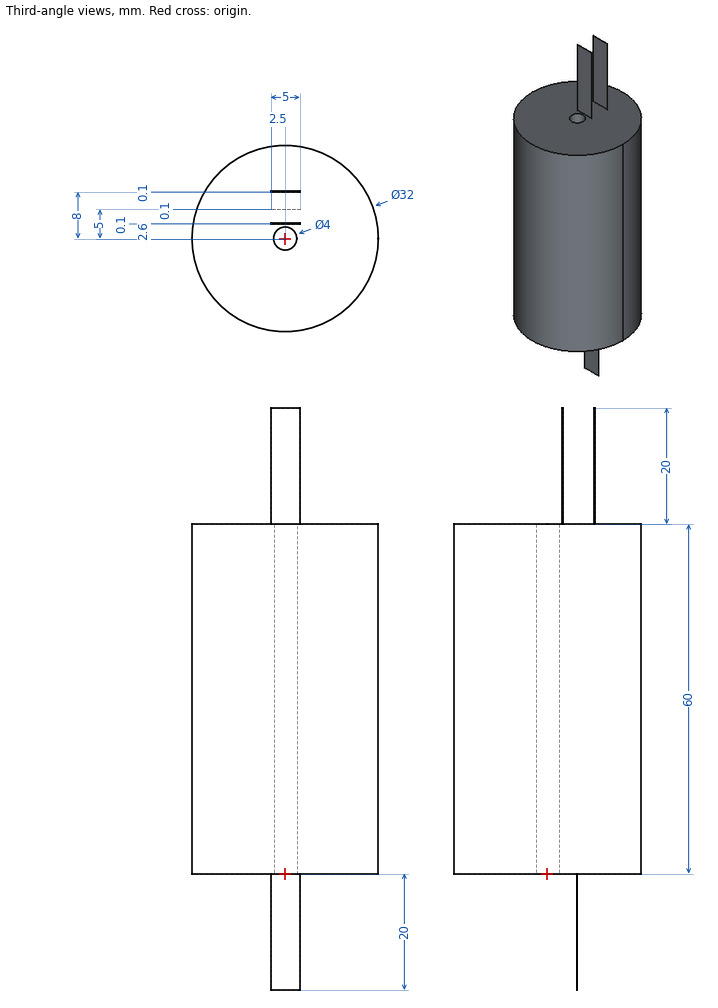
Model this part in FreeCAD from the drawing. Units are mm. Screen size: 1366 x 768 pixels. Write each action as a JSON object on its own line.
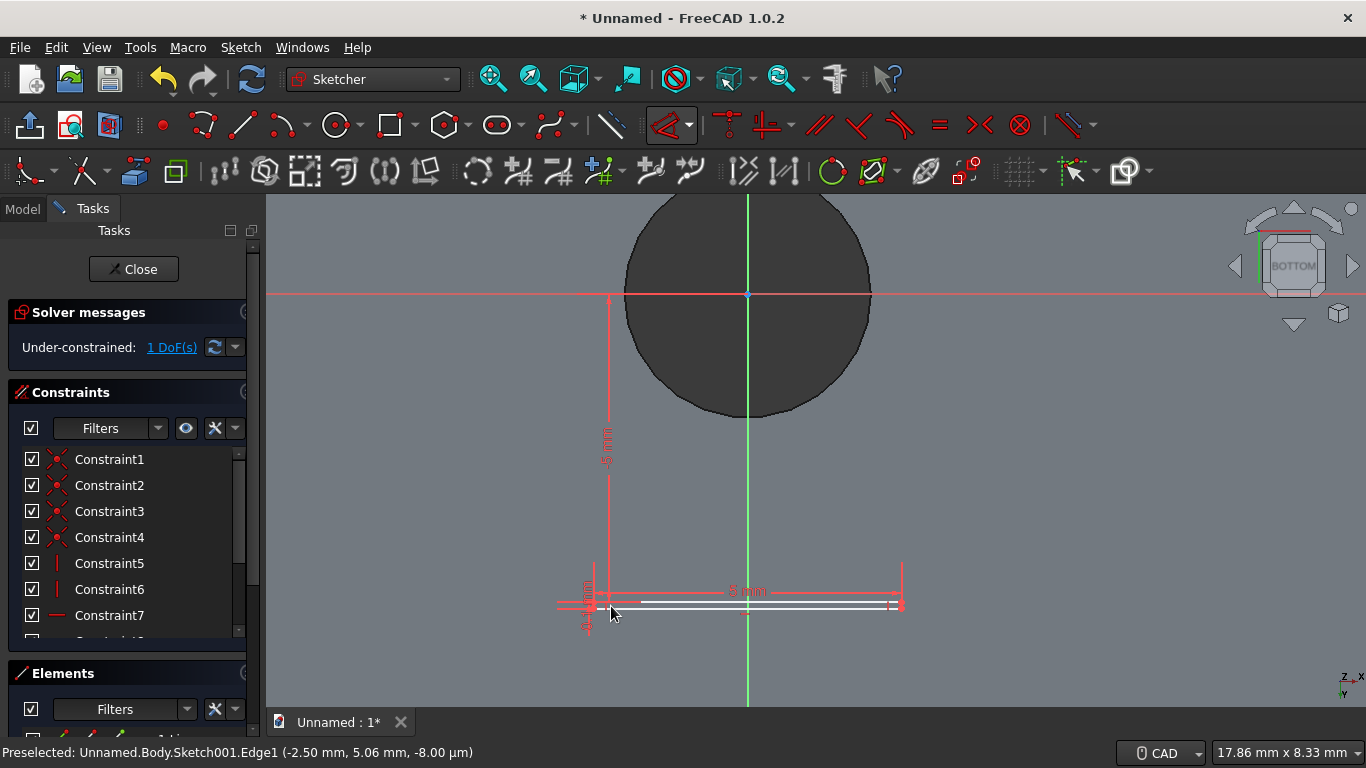
{"action": "scroll", "coordinate": [594, 602], "scroll_direction": "up", "scroll_amount": 4}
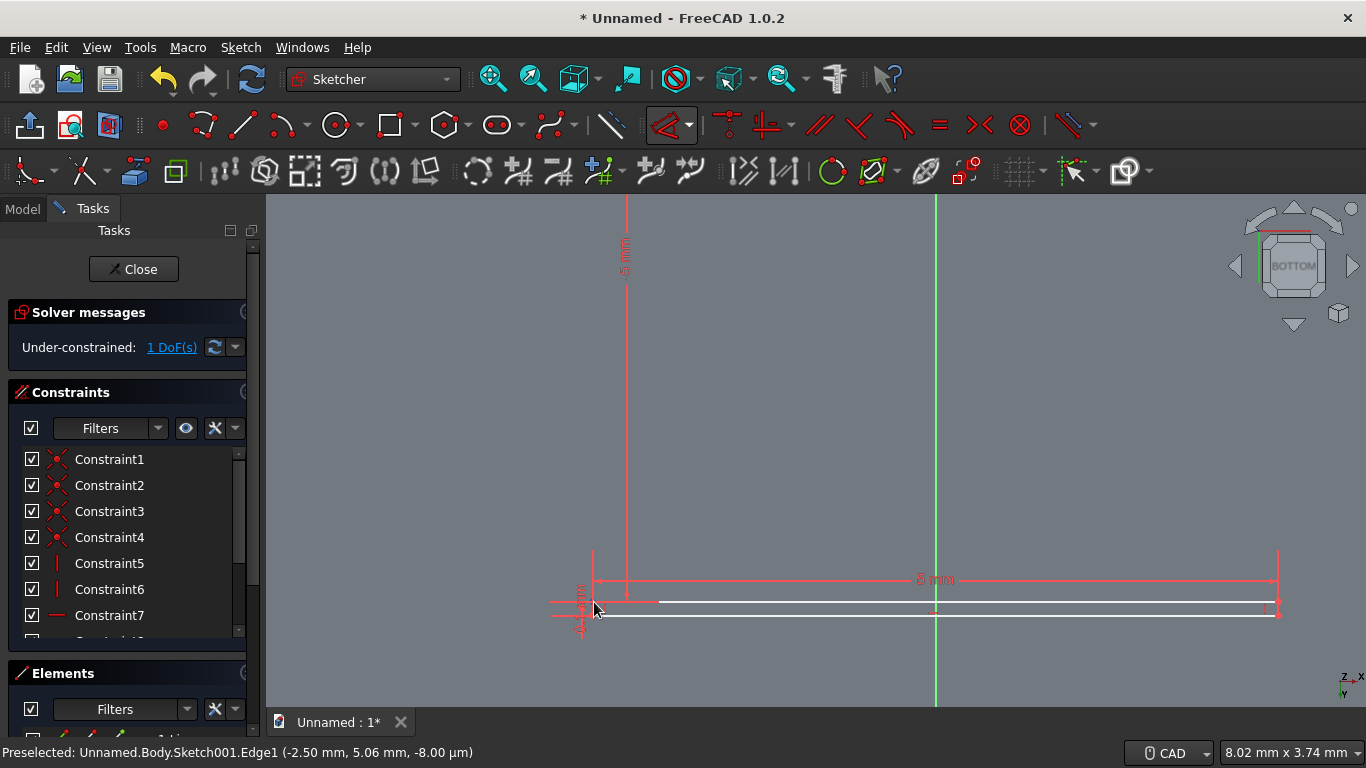
{"action": "left_click", "coordinate": [593, 602]}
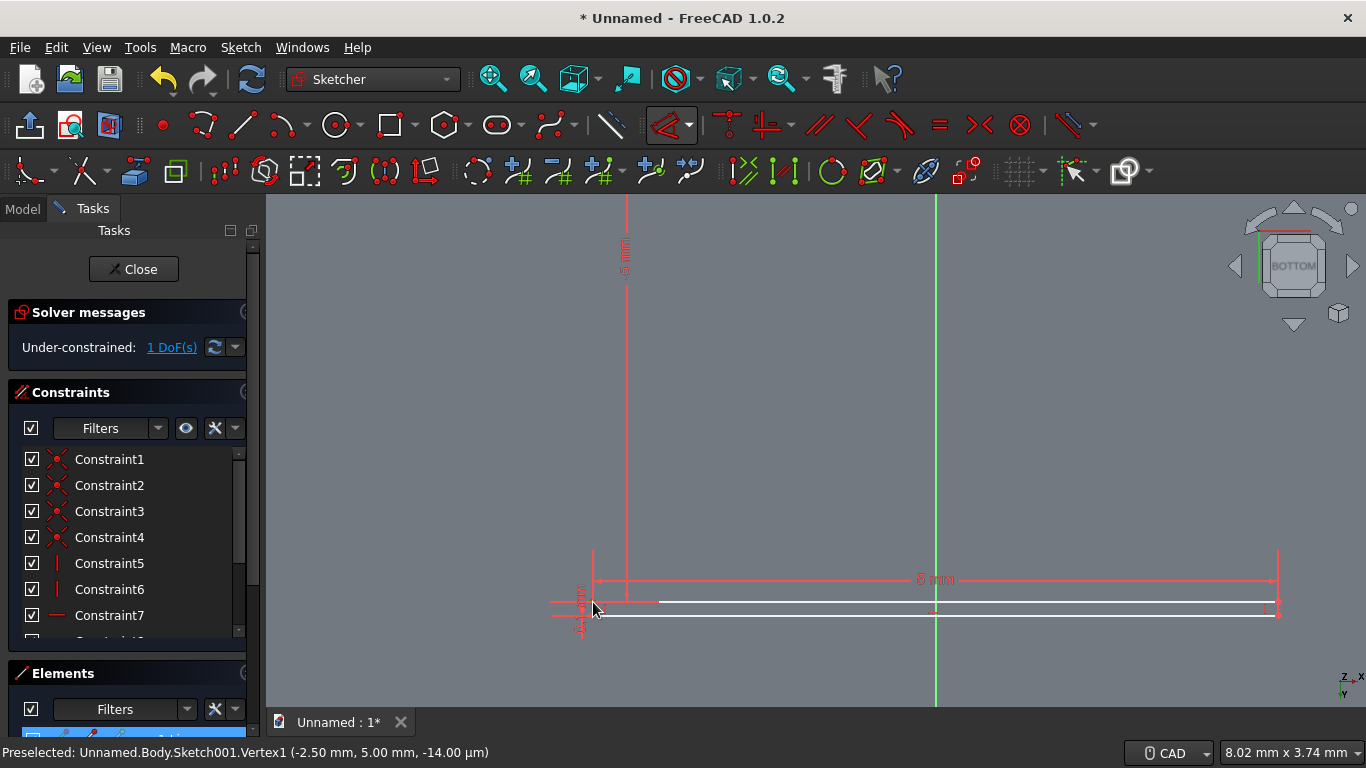
{"action": "key", "text": "l"}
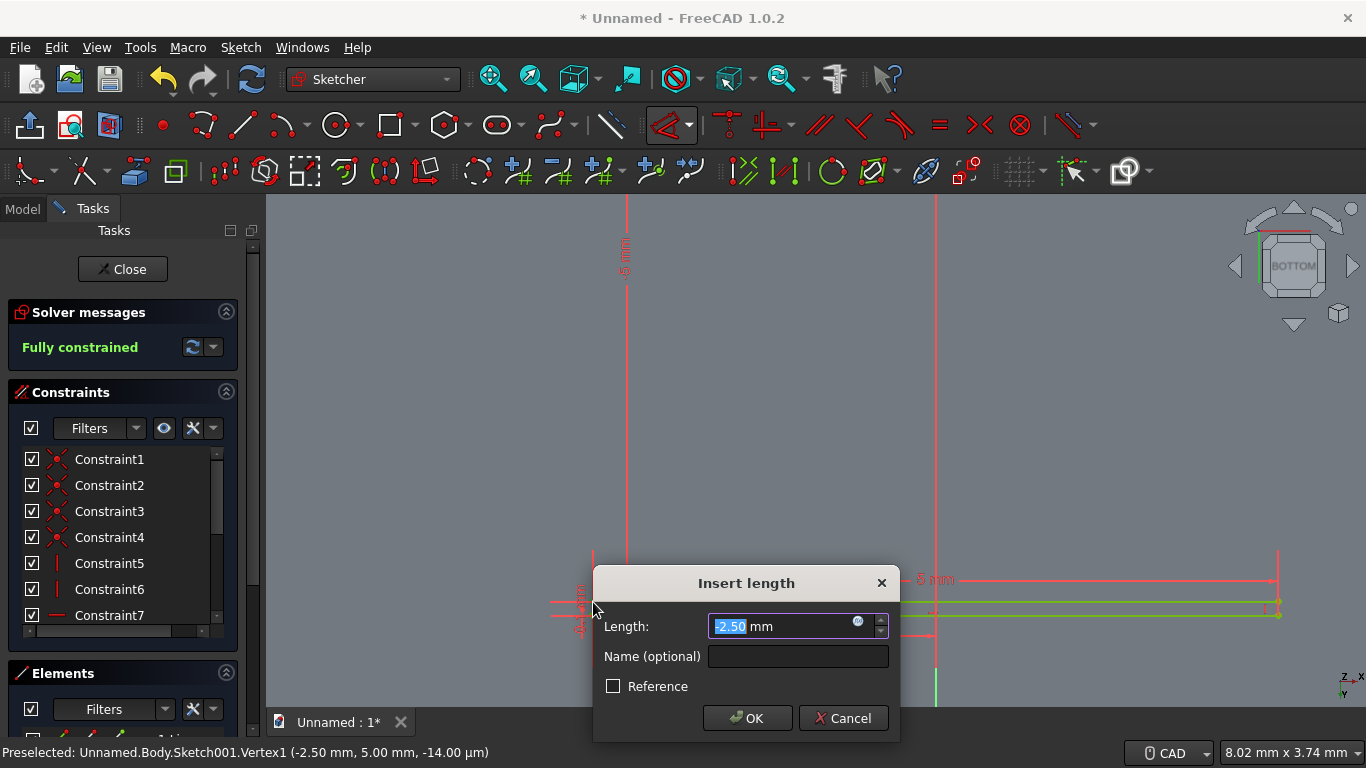
{"action": "type", "text": "-2.5"}
{"action": "key", "text": "Return"}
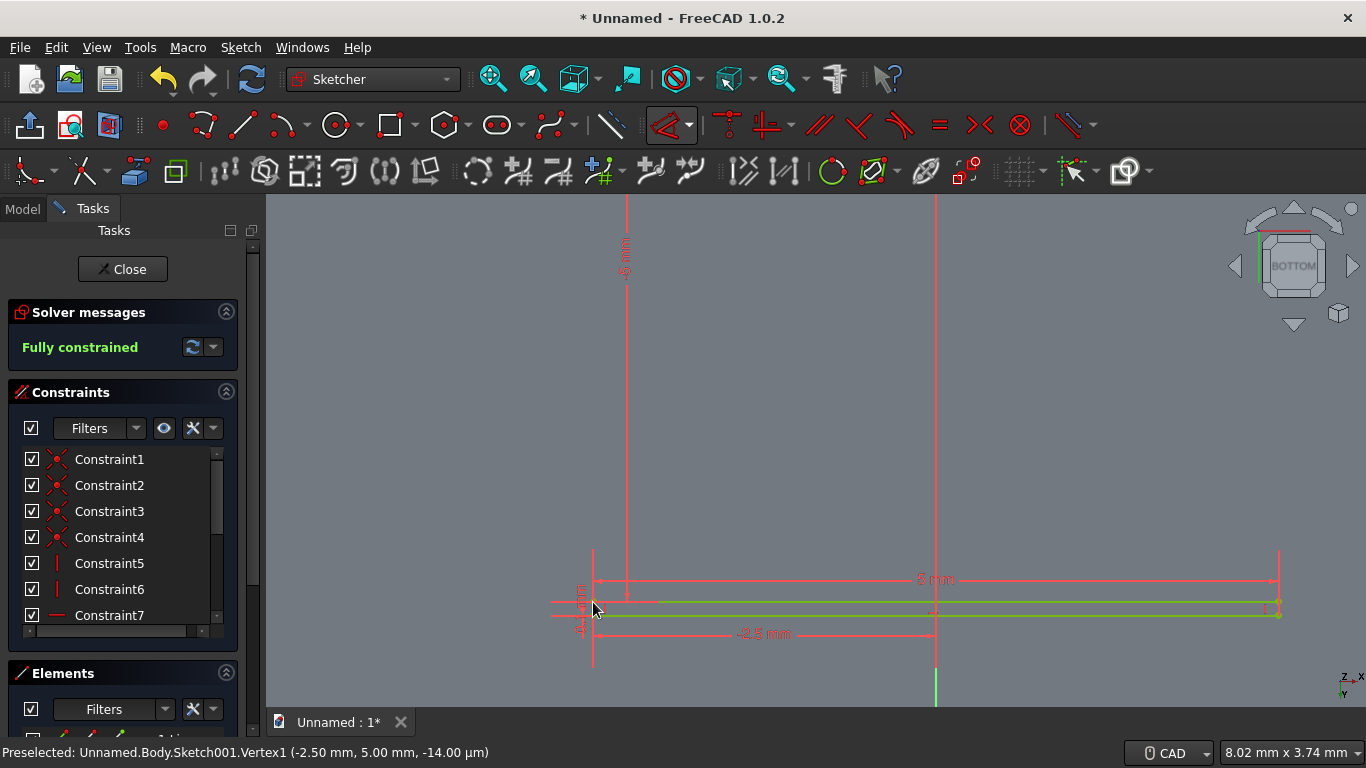
{"action": "left_click", "coordinate": [123, 269]}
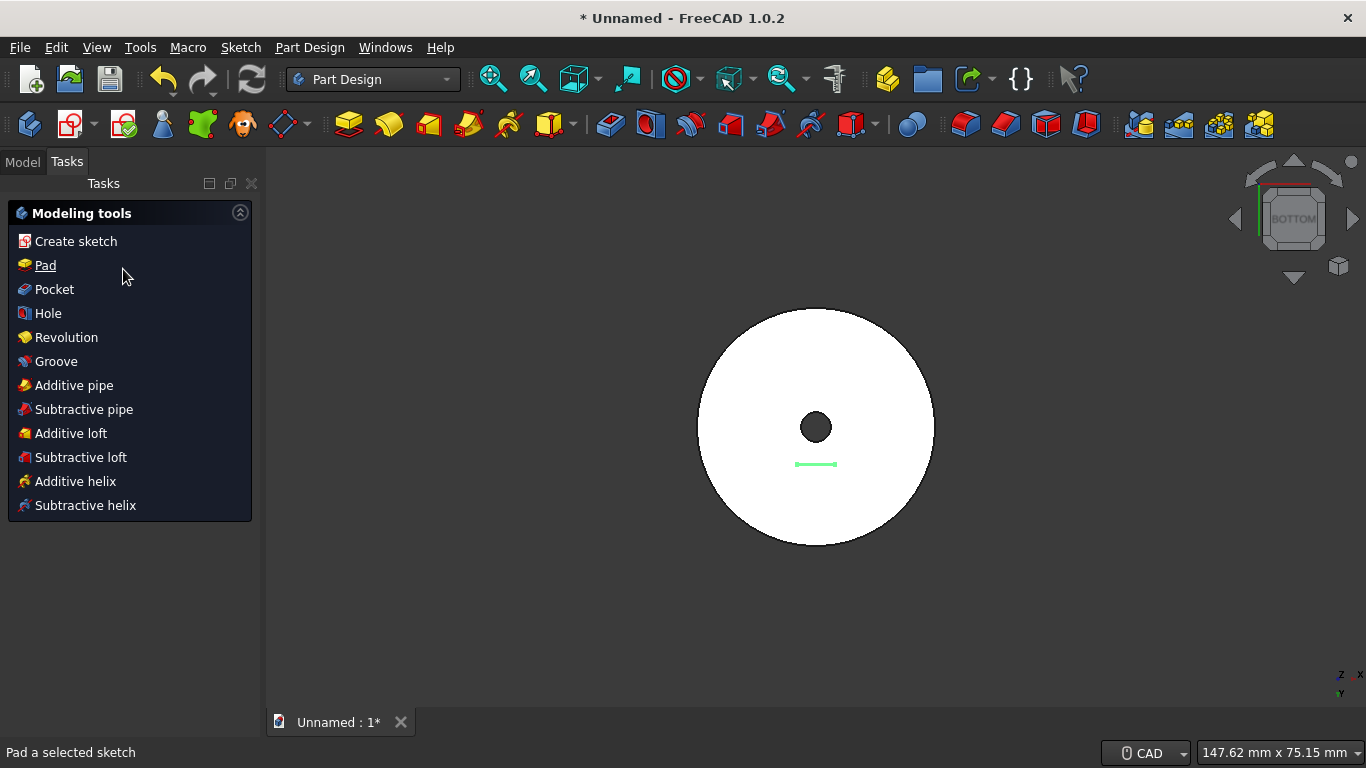
{"action": "left_click", "coordinate": [350, 124]}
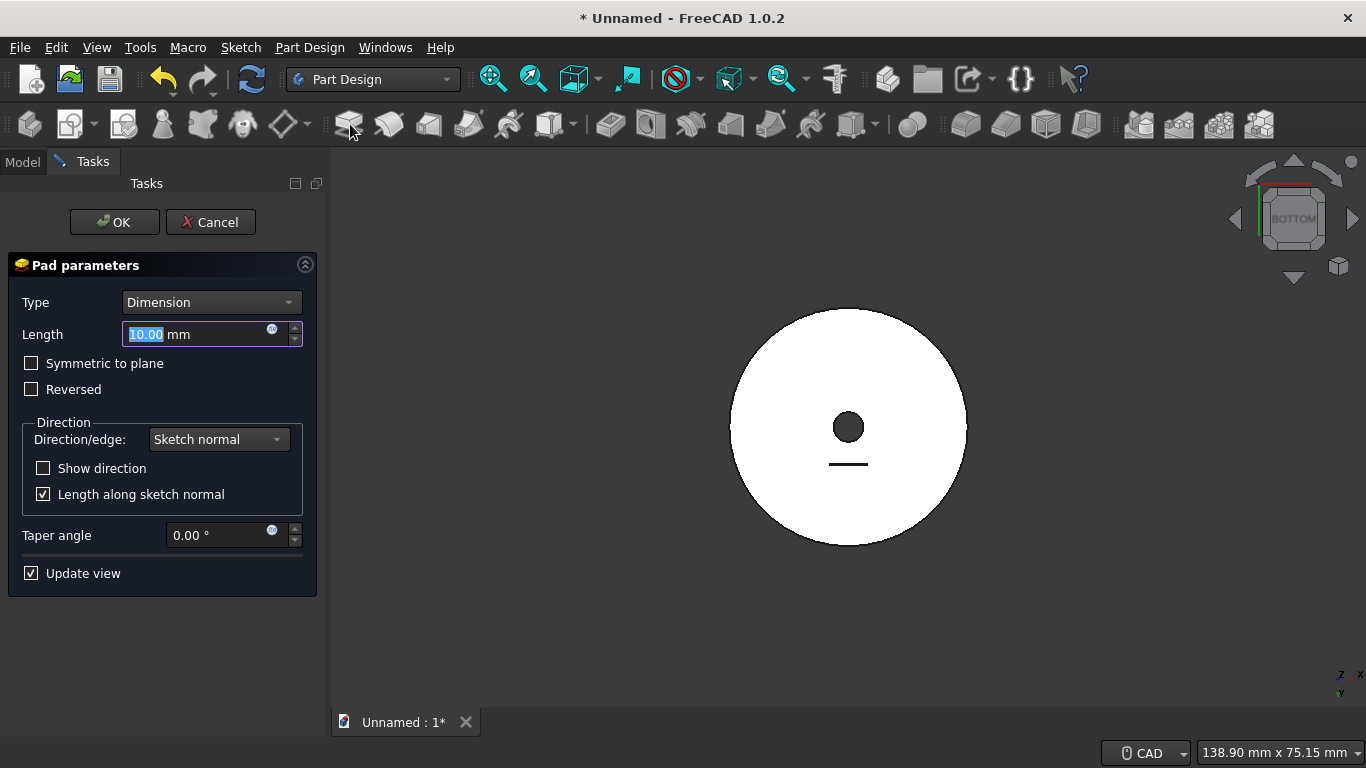
{"action": "type", "text": "20"}
{"action": "key", "text": "Tab"}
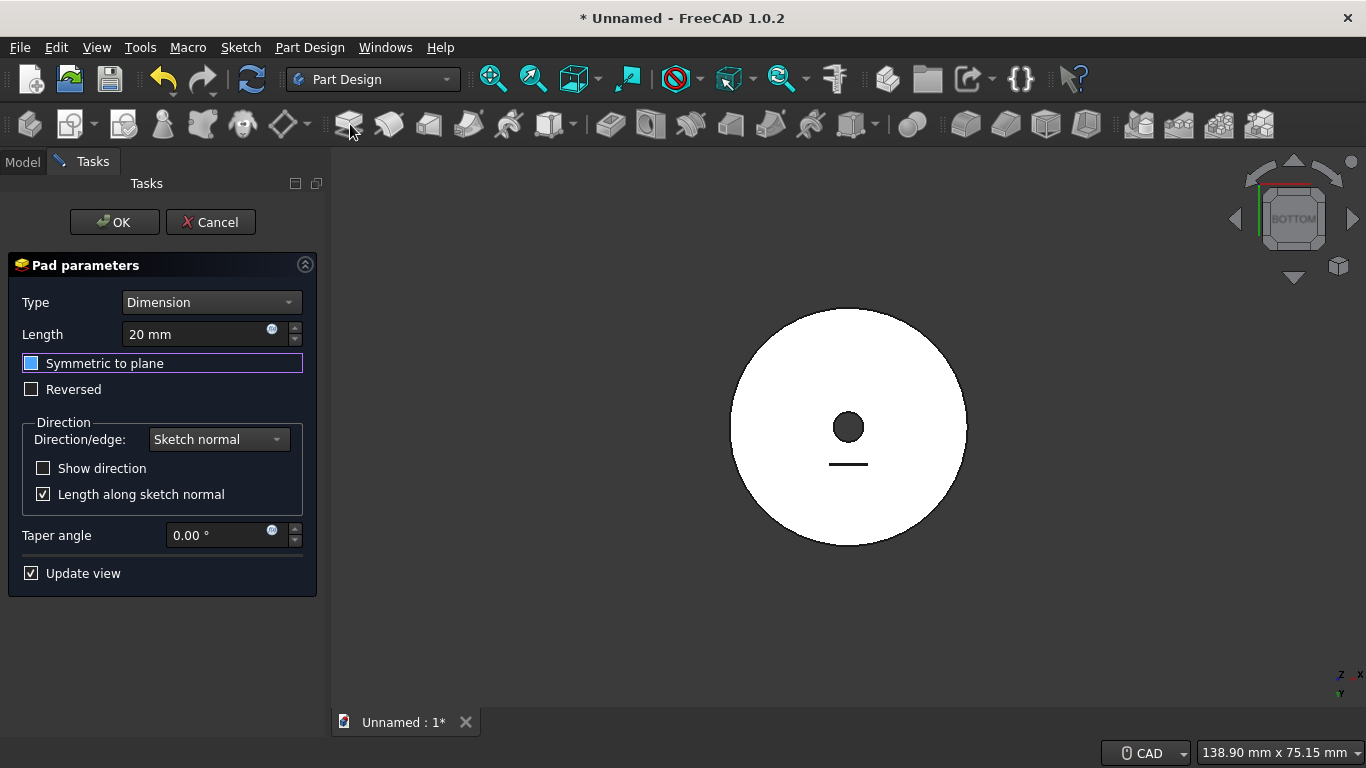
{"action": "left_click", "coordinate": [115, 222]}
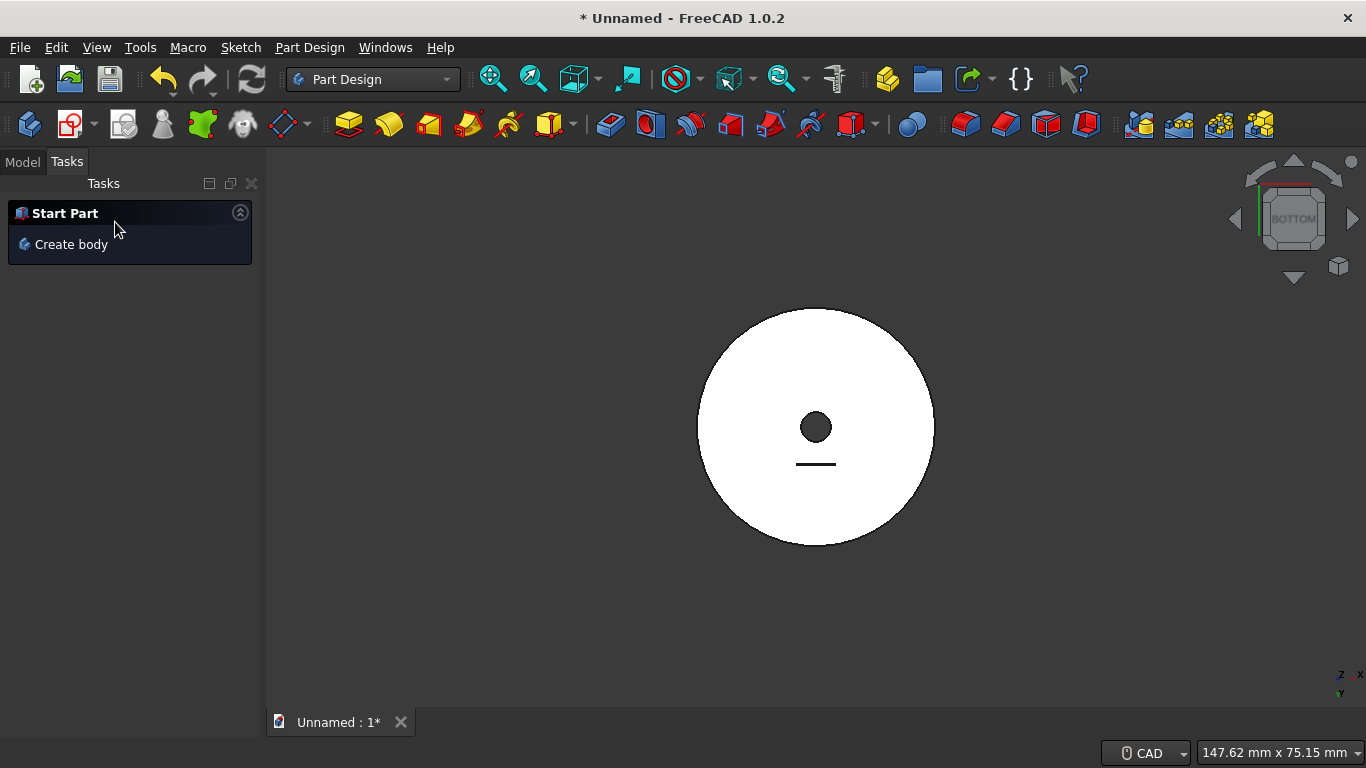
{"action": "left_click", "coordinate": [494, 80]}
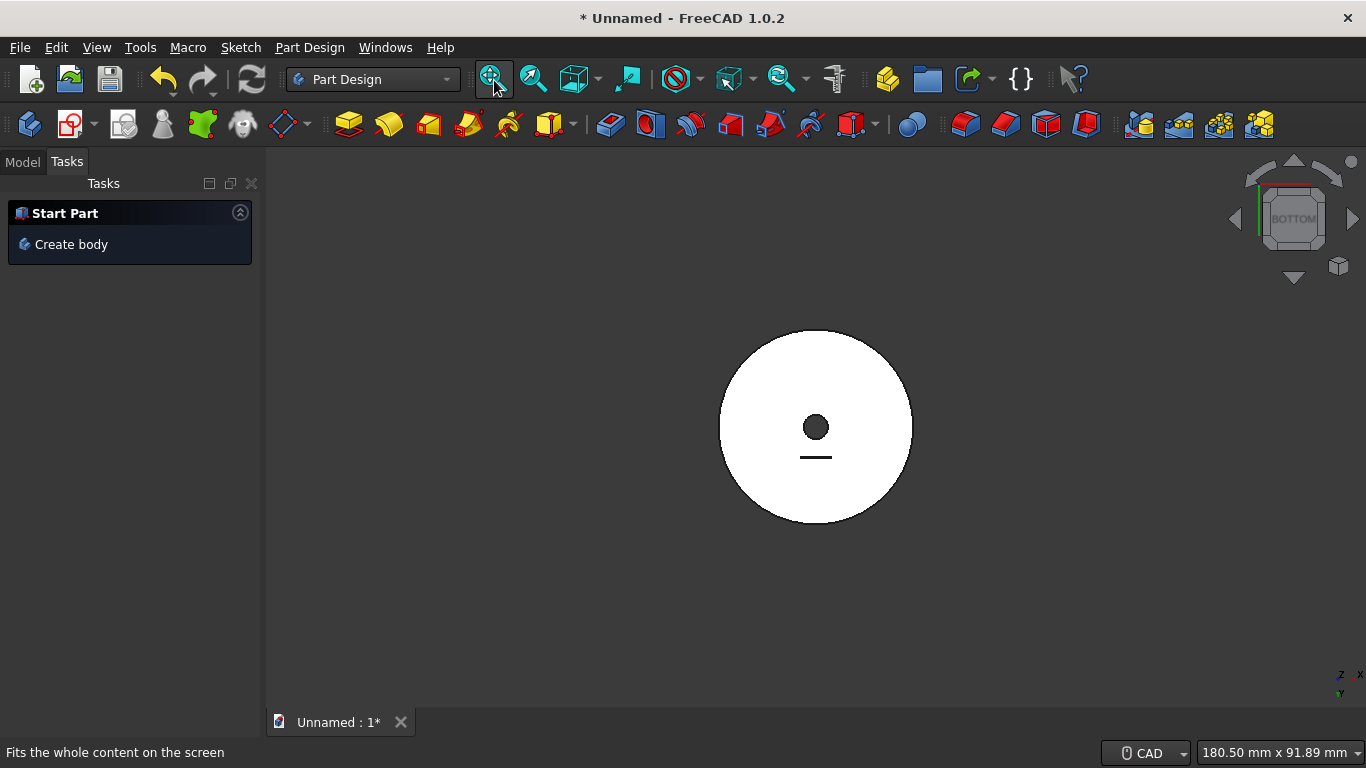
{"action": "key", "text": "0"}